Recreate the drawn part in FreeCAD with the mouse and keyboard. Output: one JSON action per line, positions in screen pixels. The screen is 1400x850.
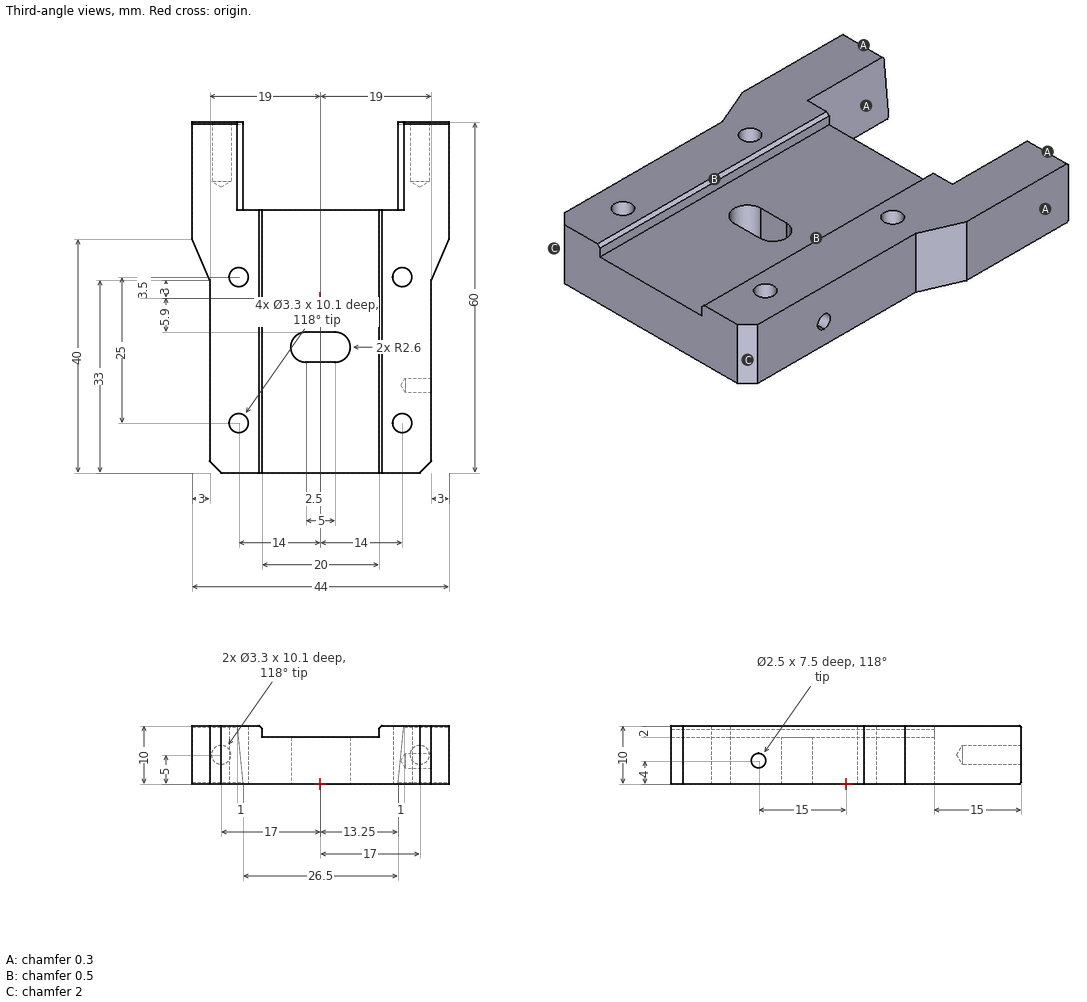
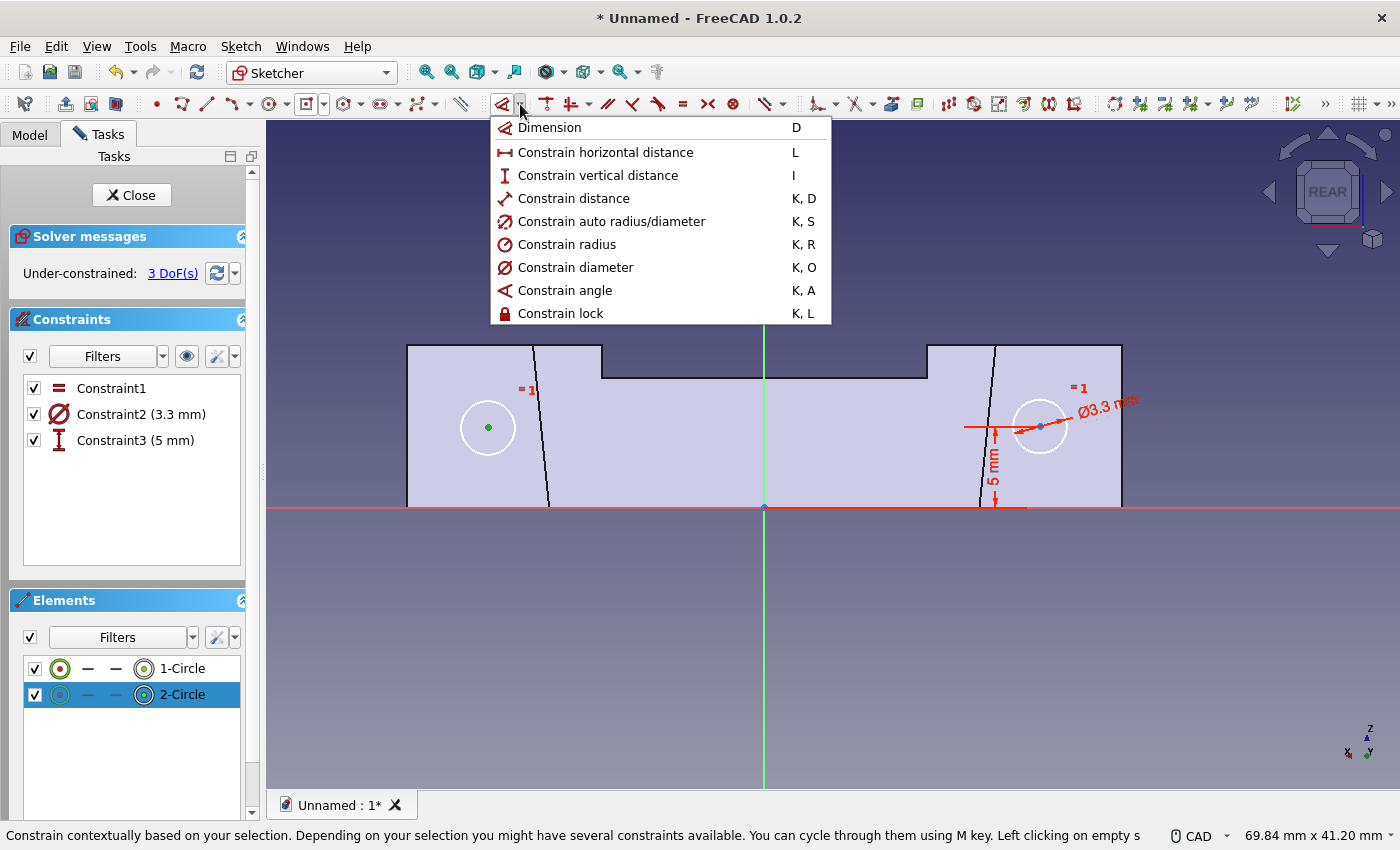
{"action": "left_click", "coordinate": [661, 176]}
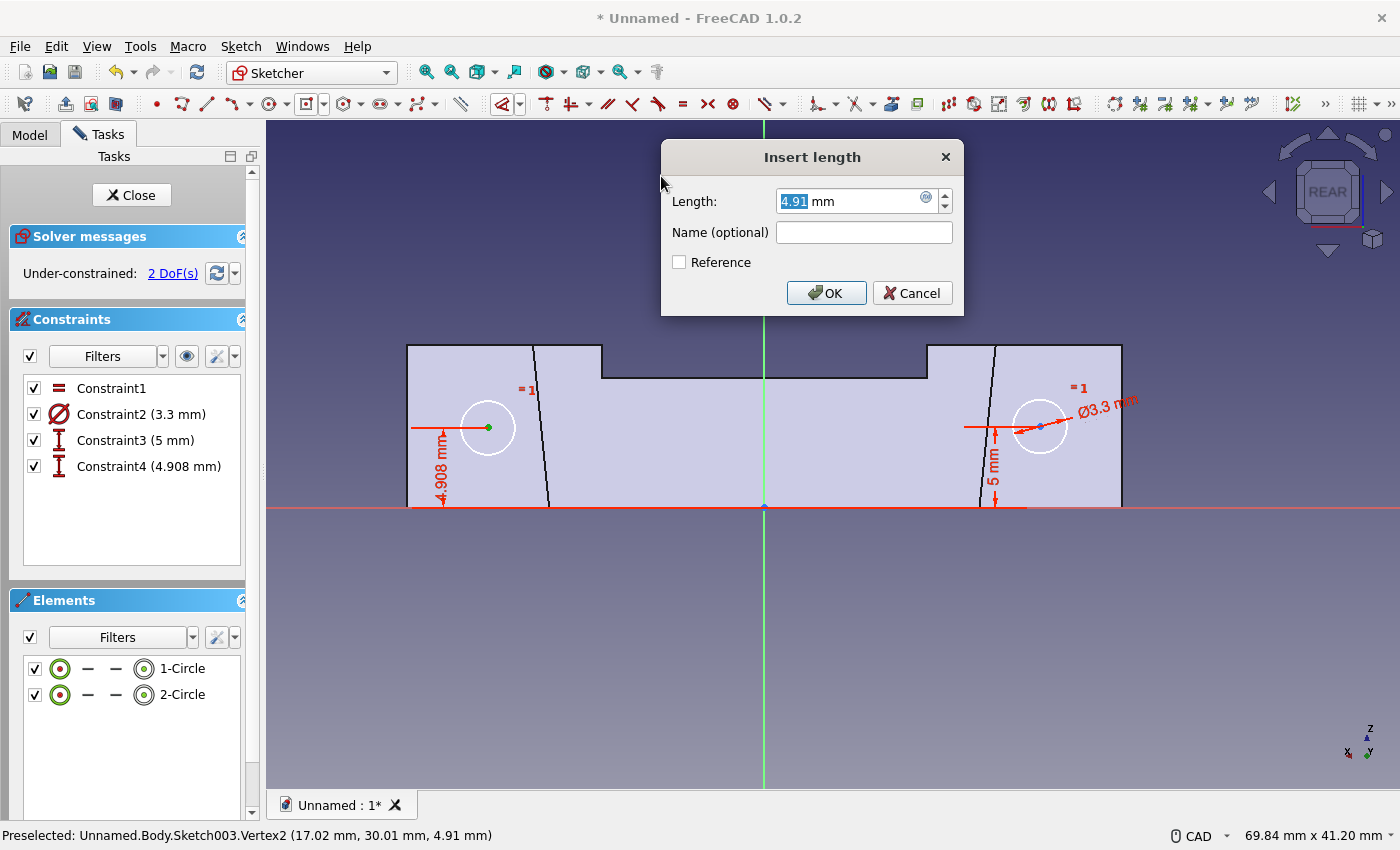
{"action": "type", "text": "5"}
{"action": "key", "text": "Return"}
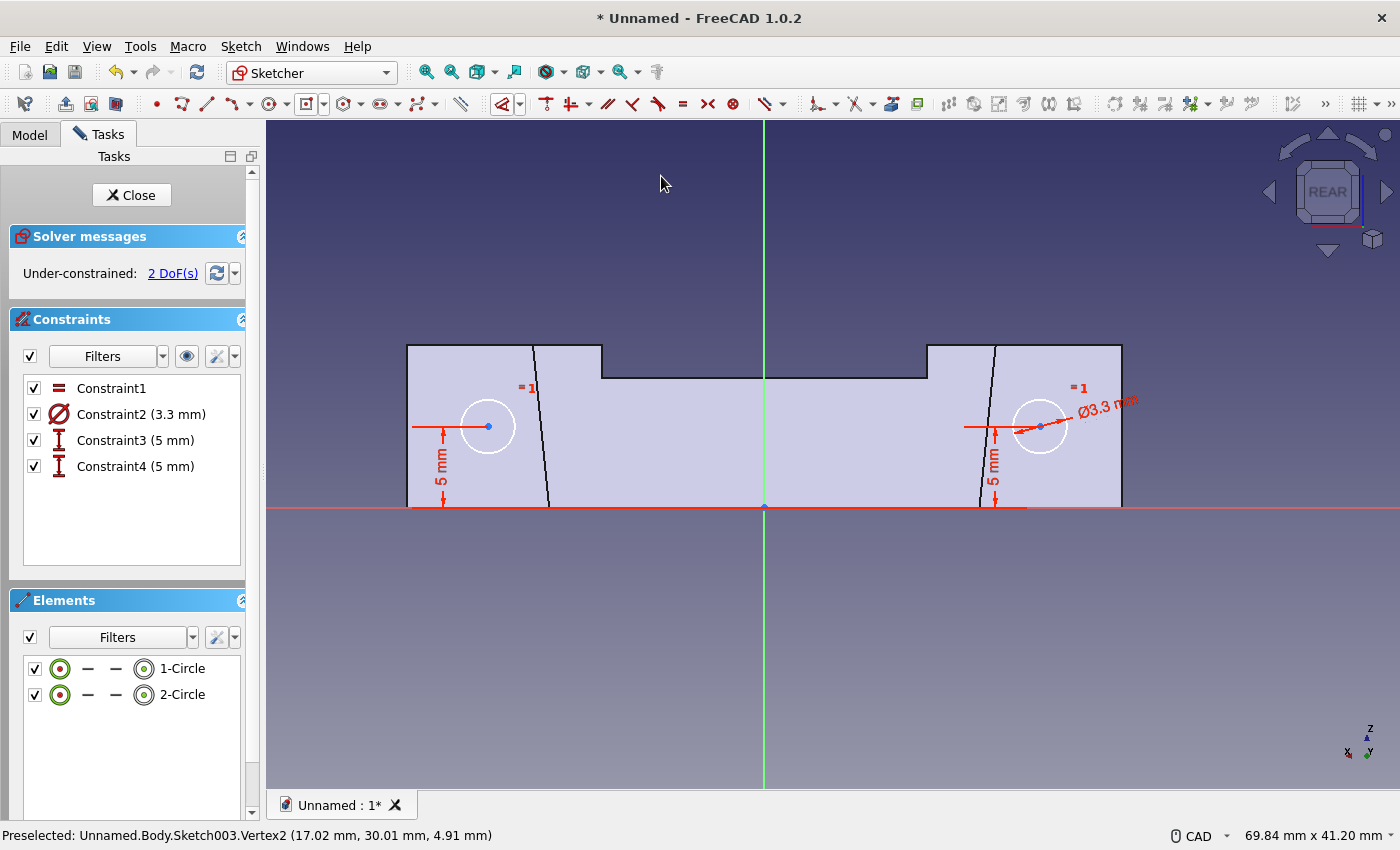
{"action": "left_click", "coordinate": [1040, 427]}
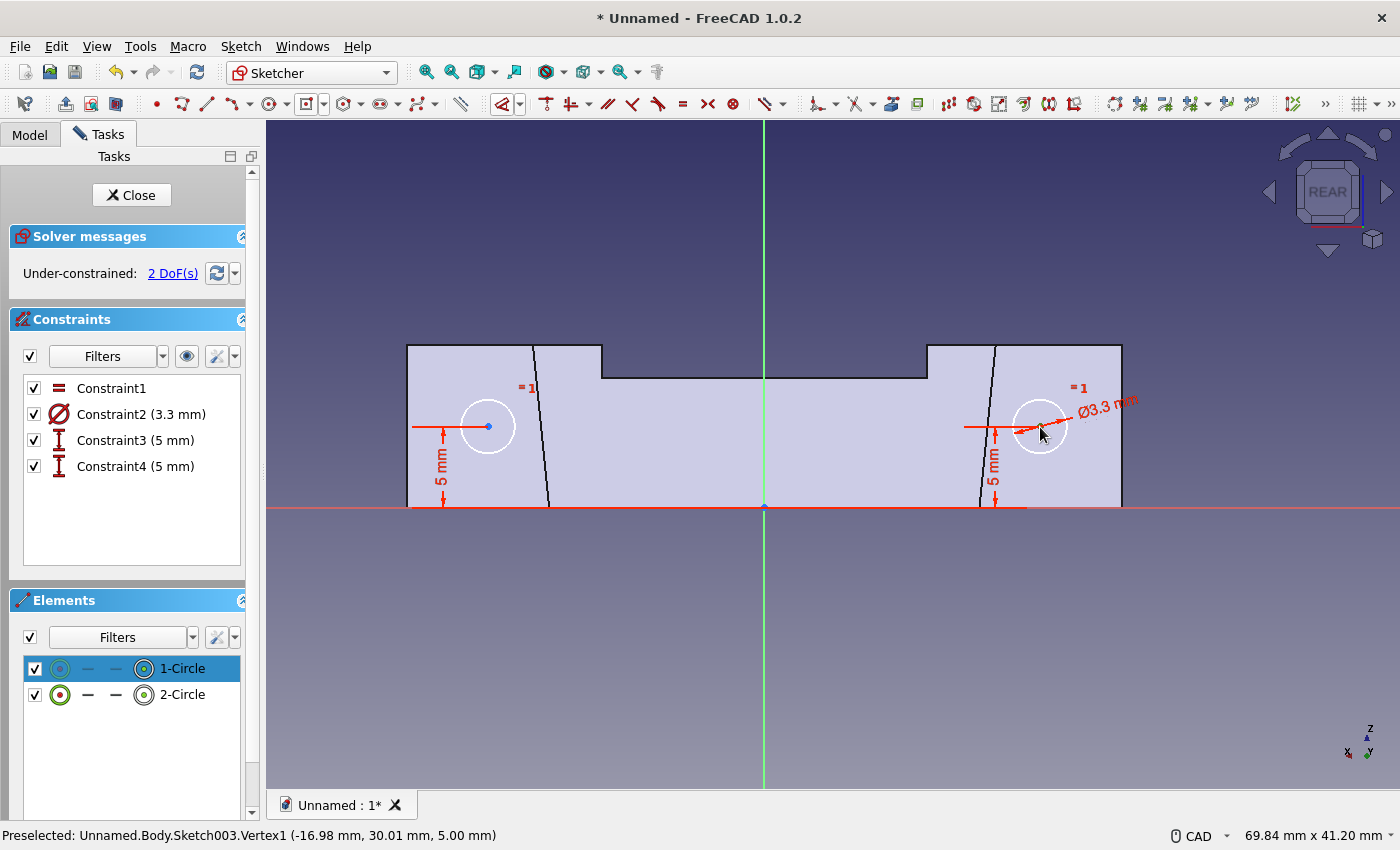
{"action": "key", "text": "l"}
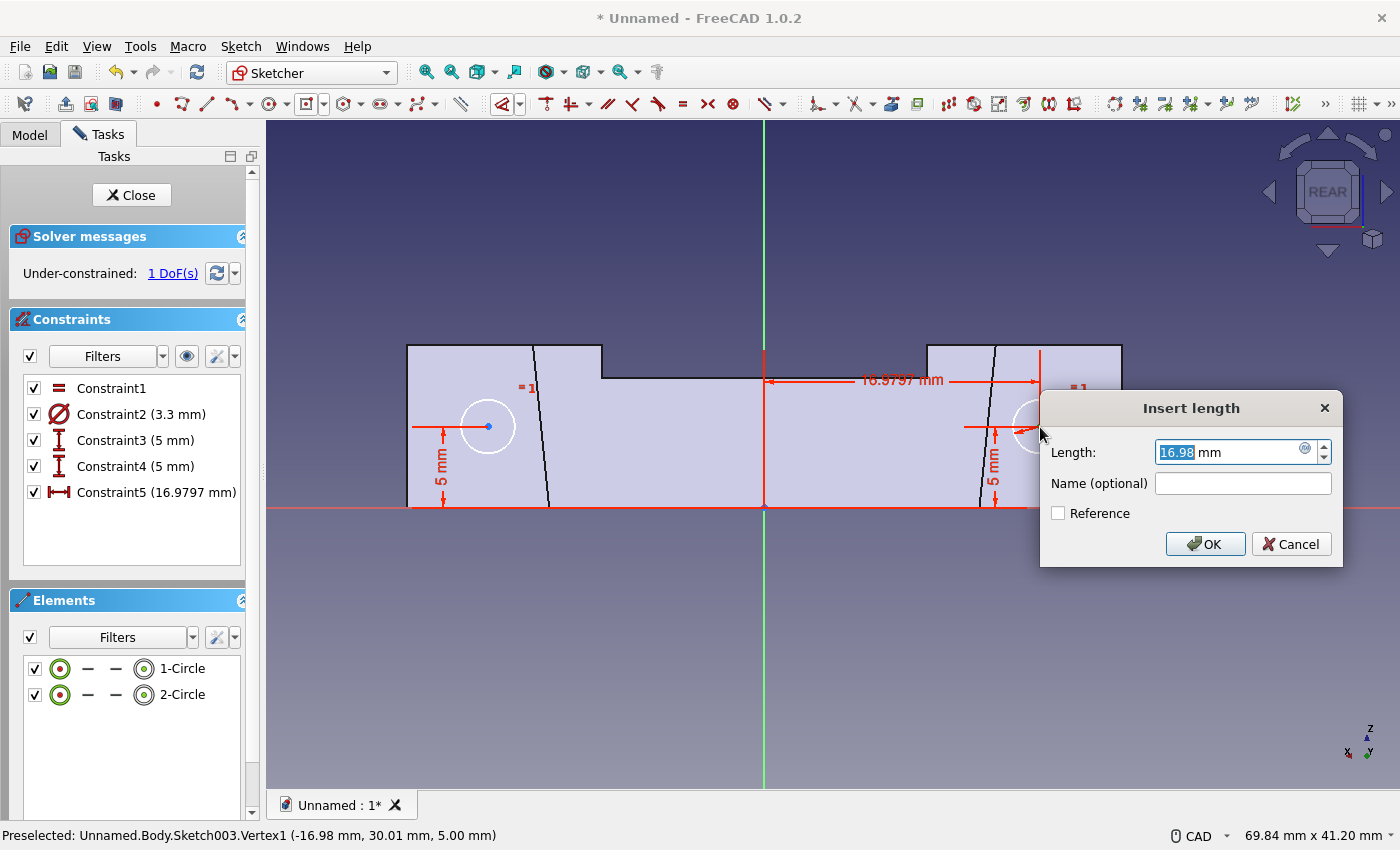
{"action": "type", "text": "17"}
{"action": "key", "text": "Return"}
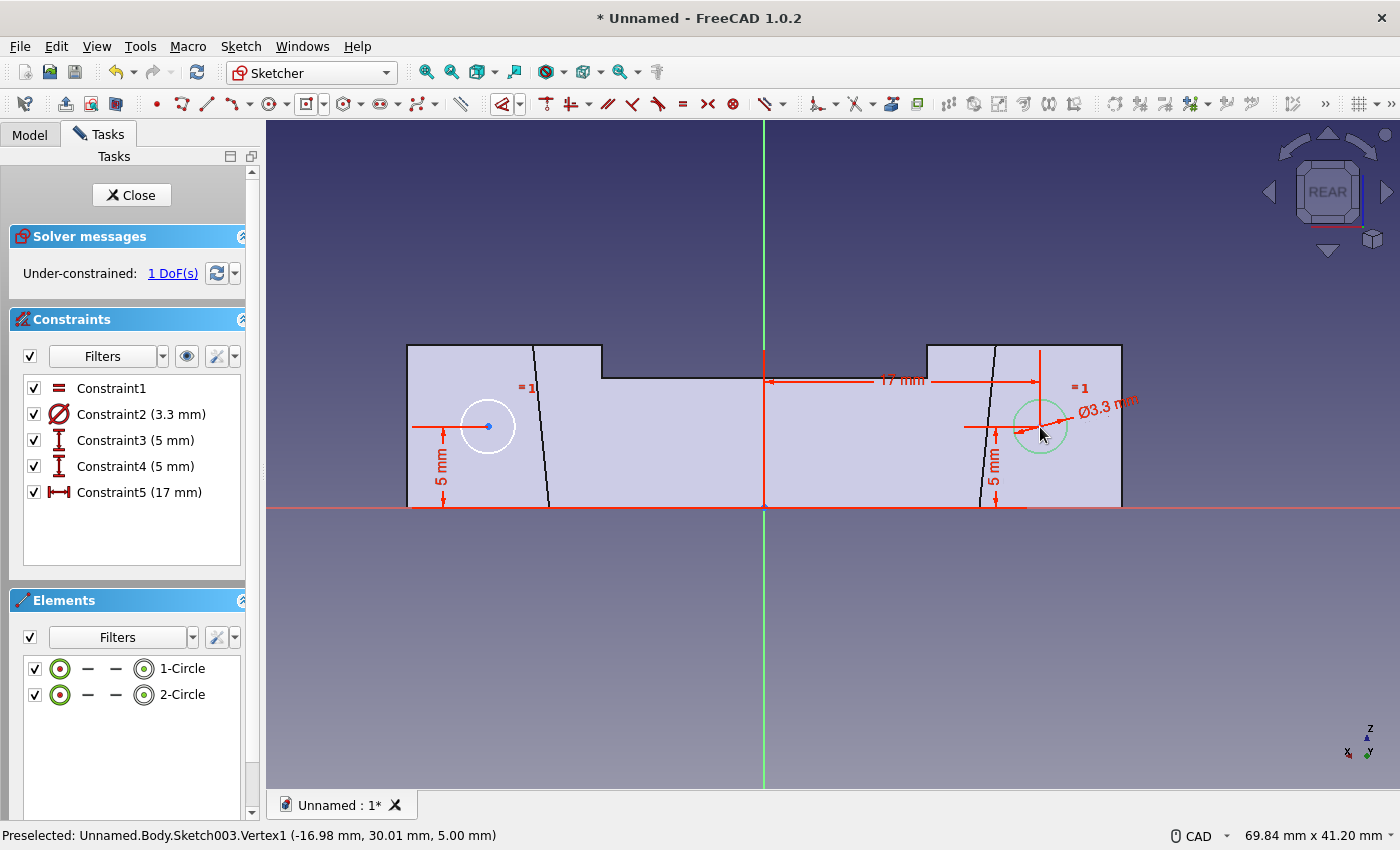
{"action": "left_click", "coordinate": [488, 427]}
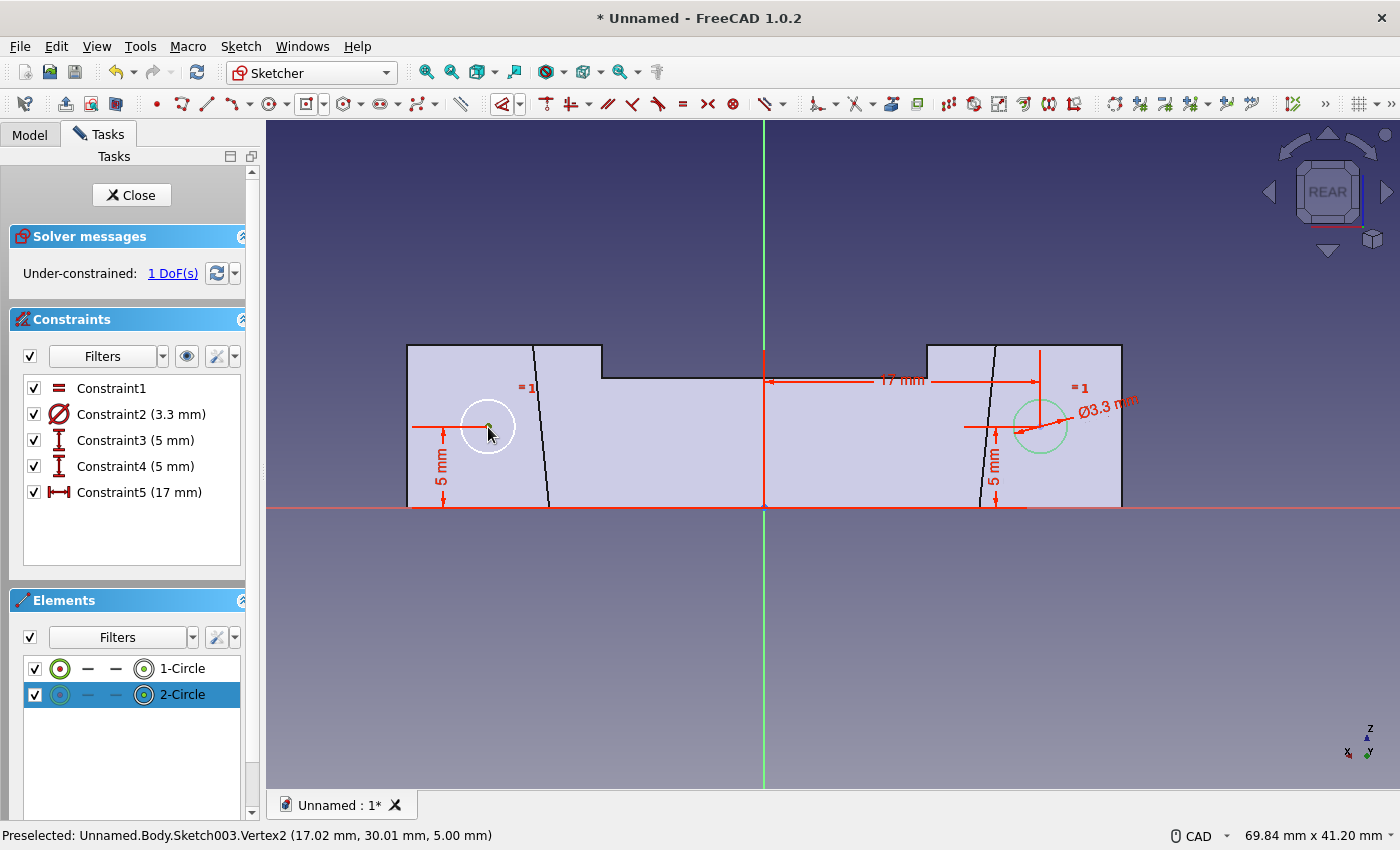
{"action": "key", "text": "l"}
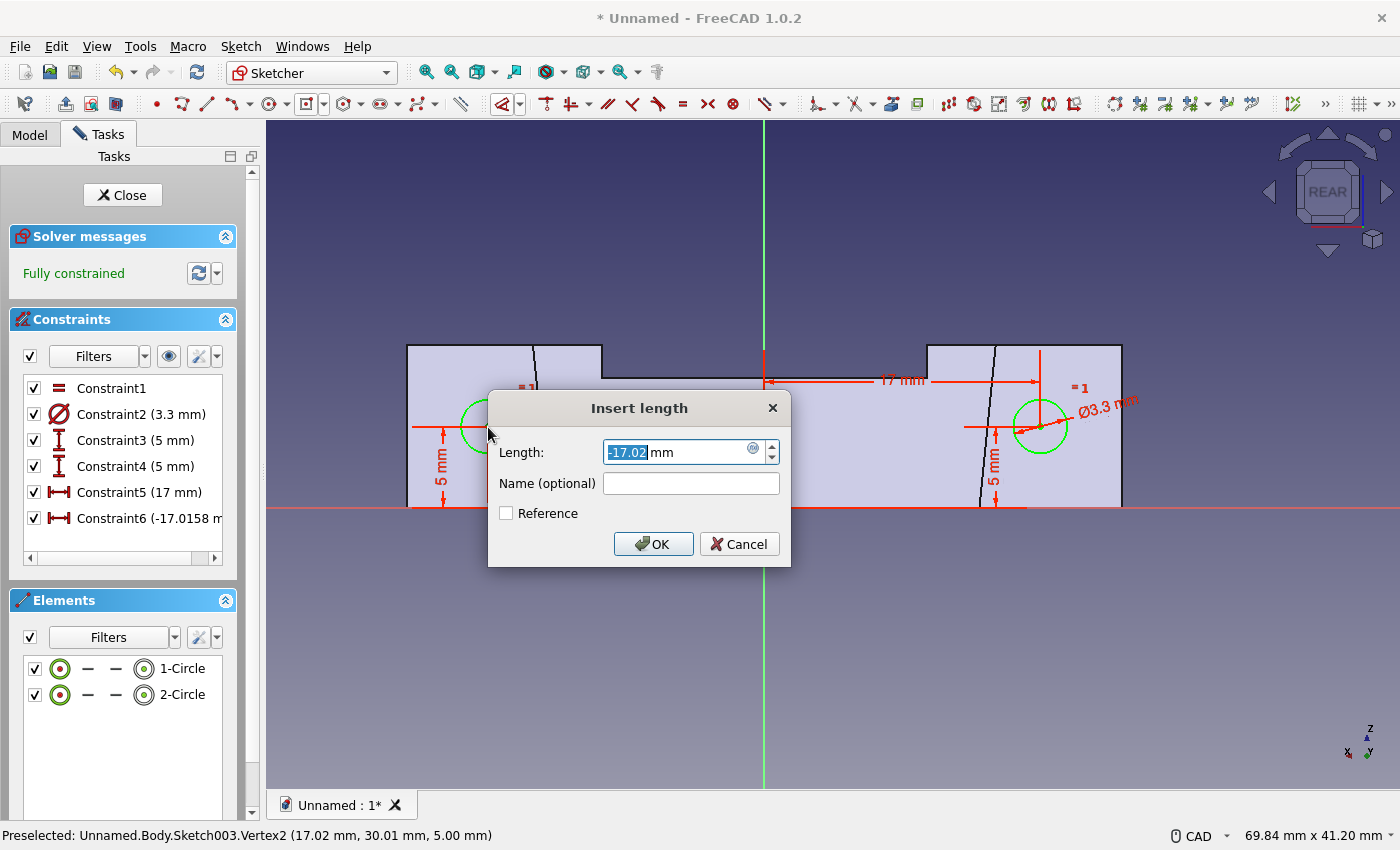
{"action": "type", "text": "-17"}
{"action": "key", "text": "Return"}